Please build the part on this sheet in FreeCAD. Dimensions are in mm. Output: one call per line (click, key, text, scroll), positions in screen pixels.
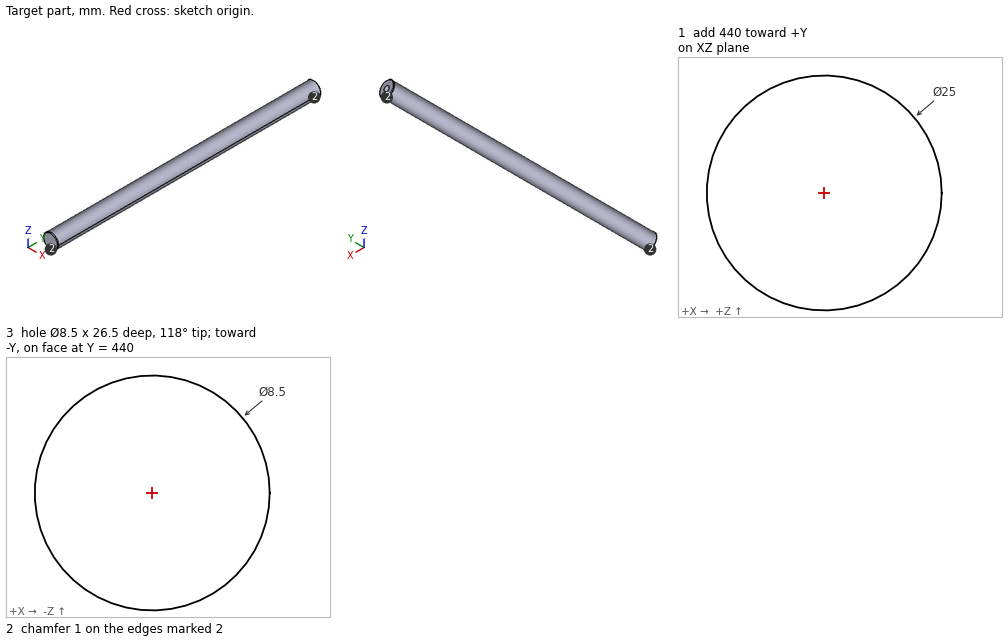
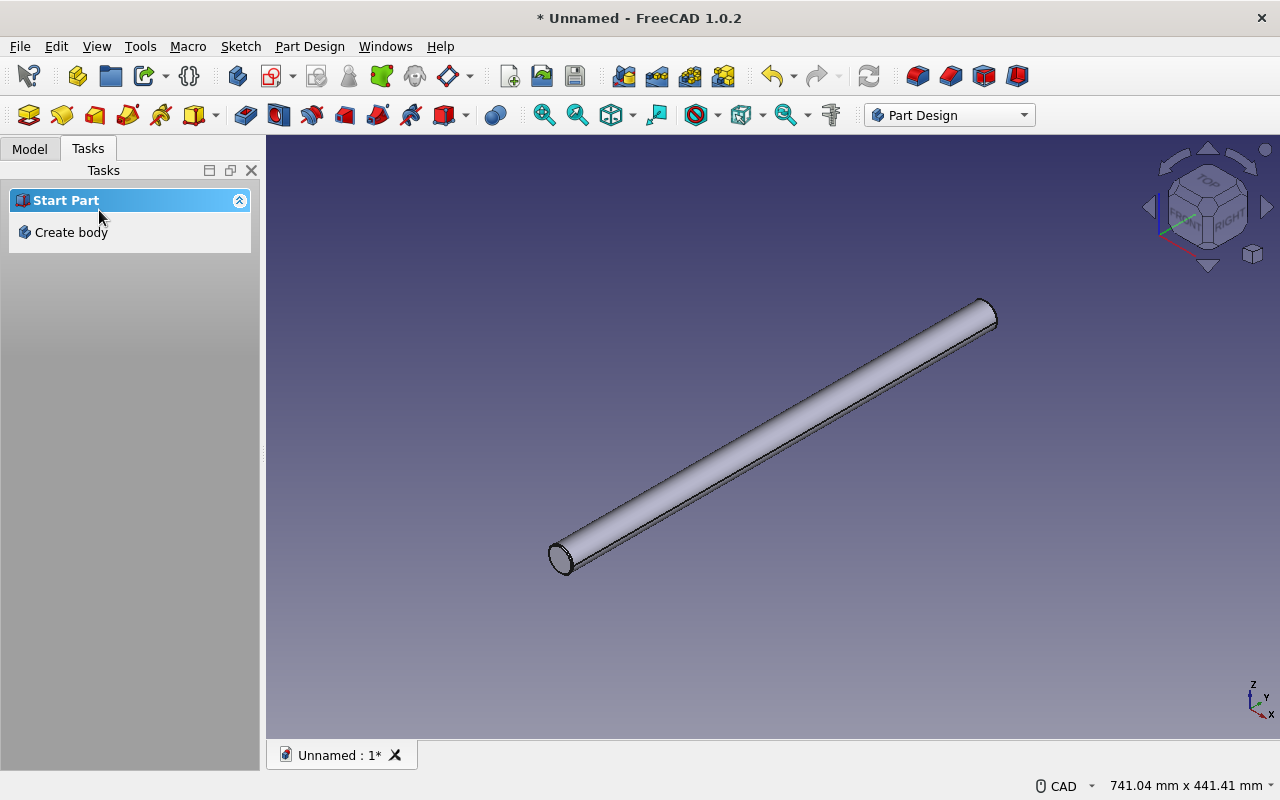
key(4)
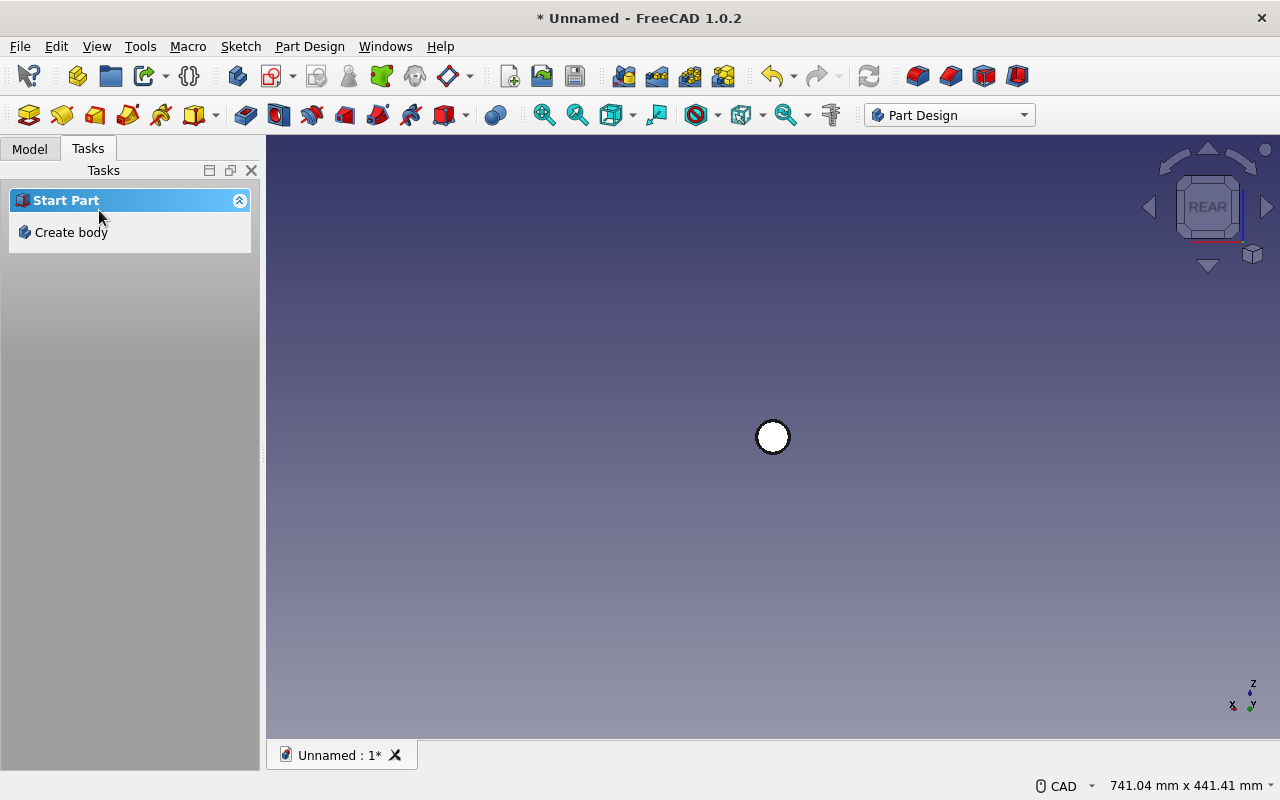
click(545, 116)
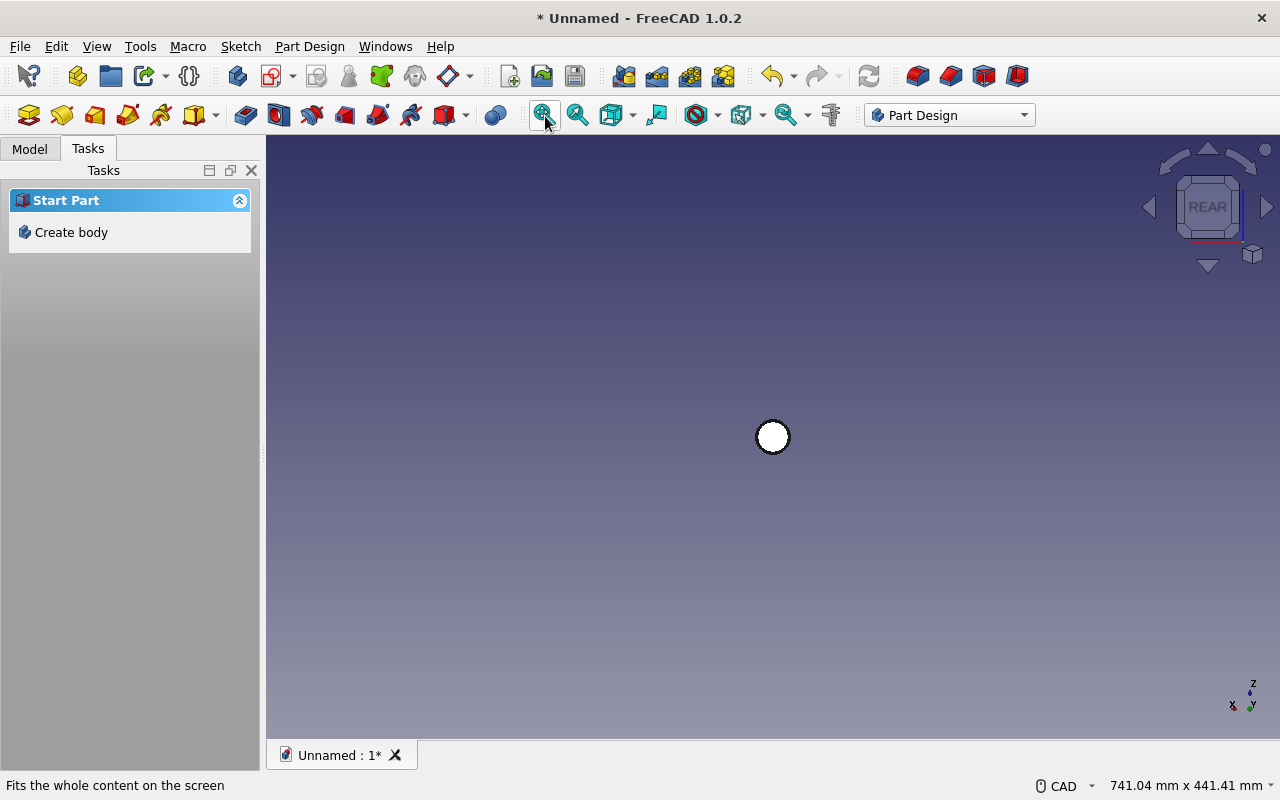
click(773, 436)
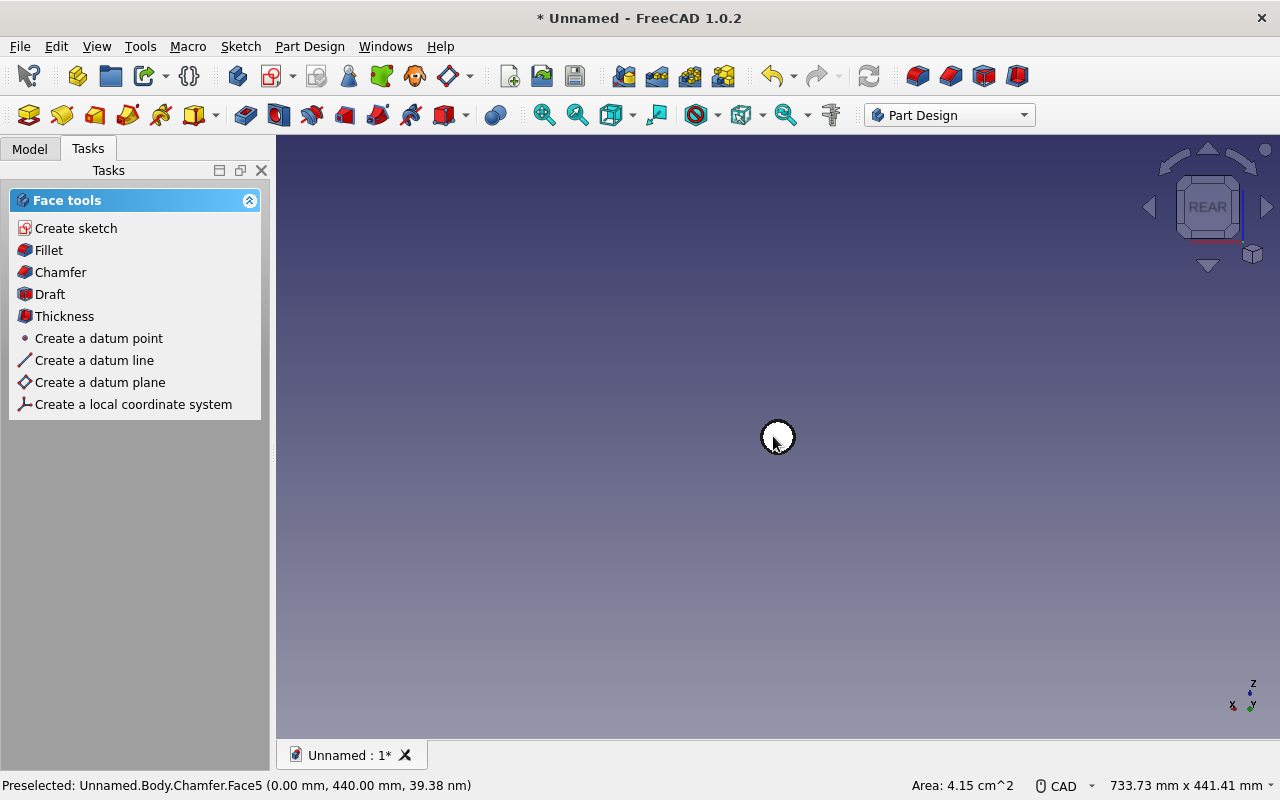
click(270, 76)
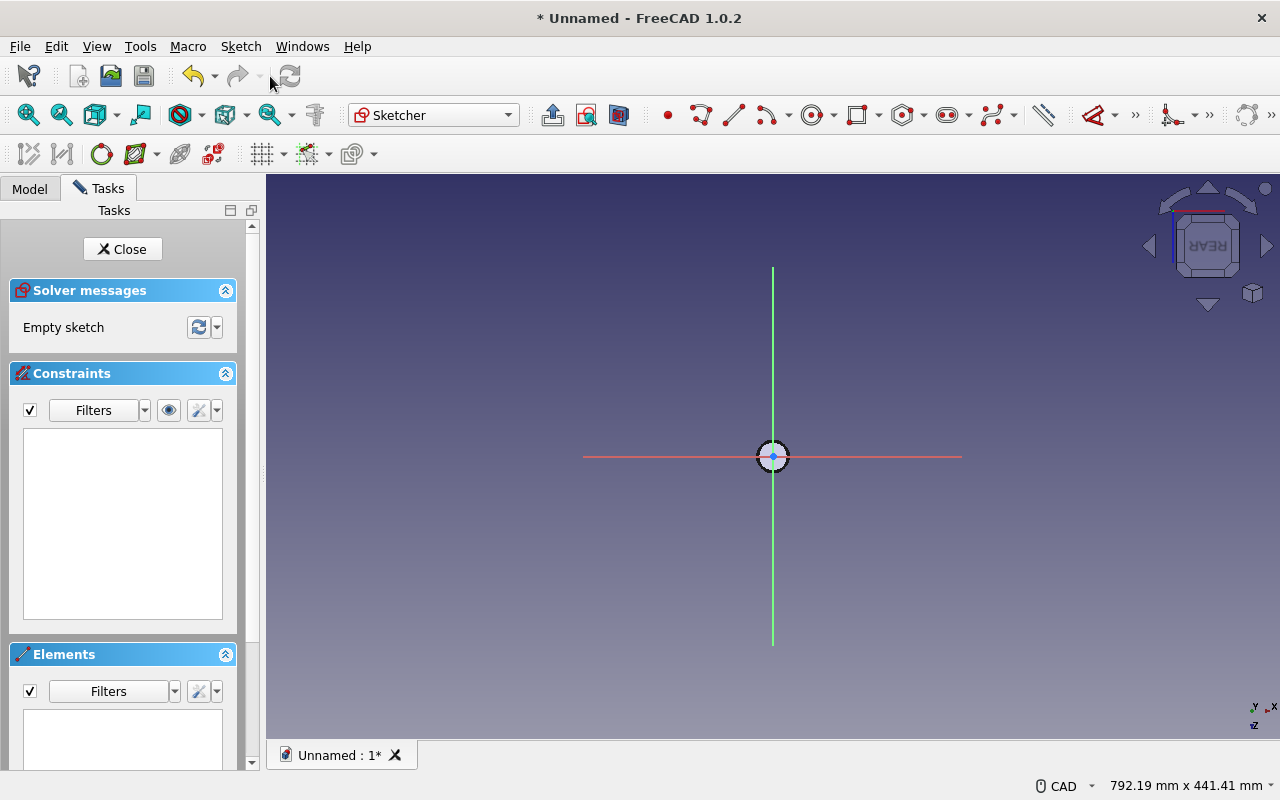
scroll(777, 456, up, 15)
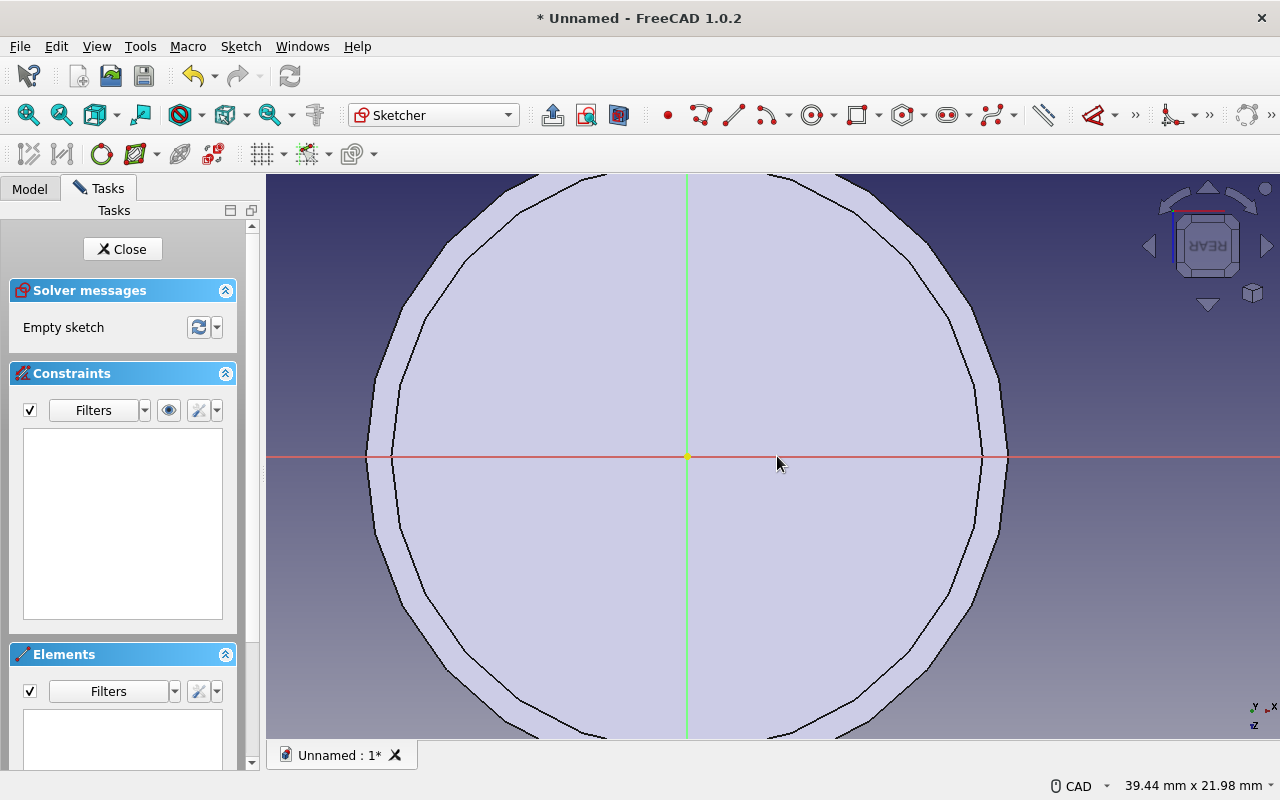
scroll(652, 456, up, 2)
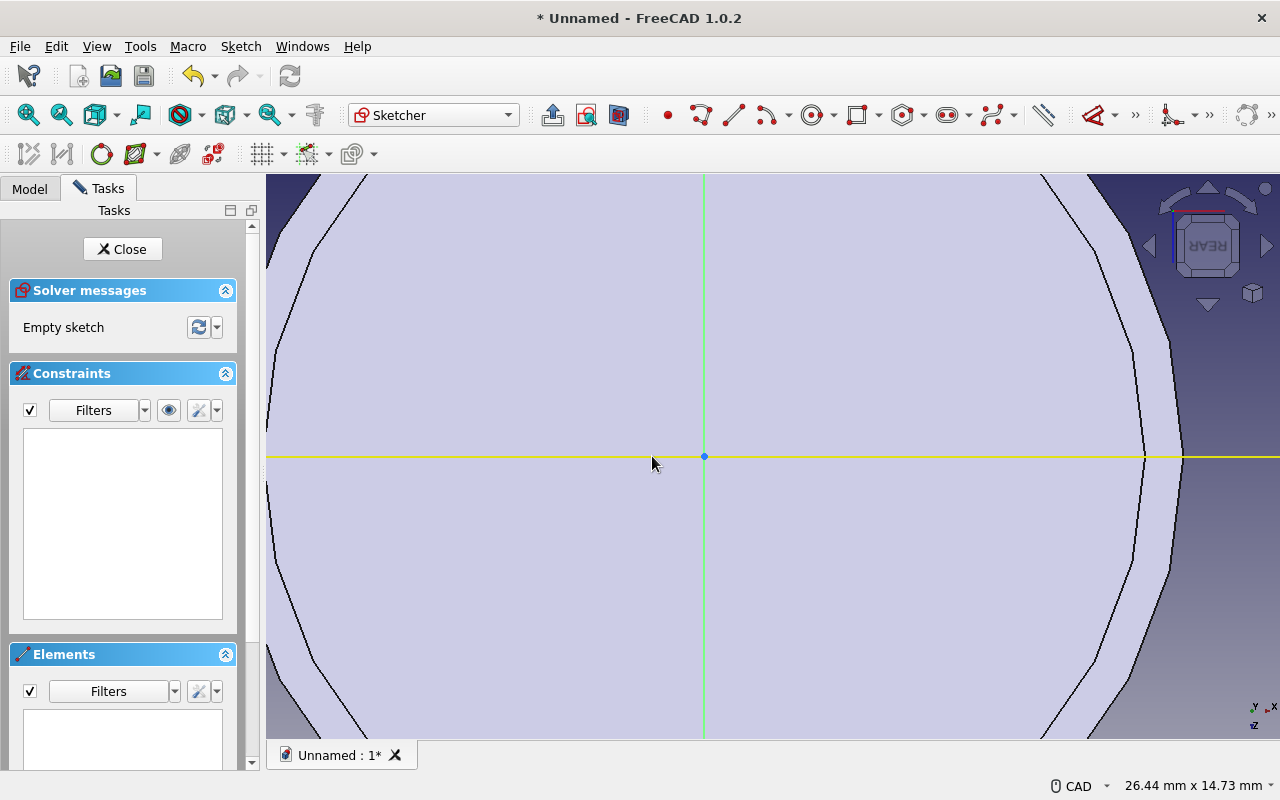
click(812, 116)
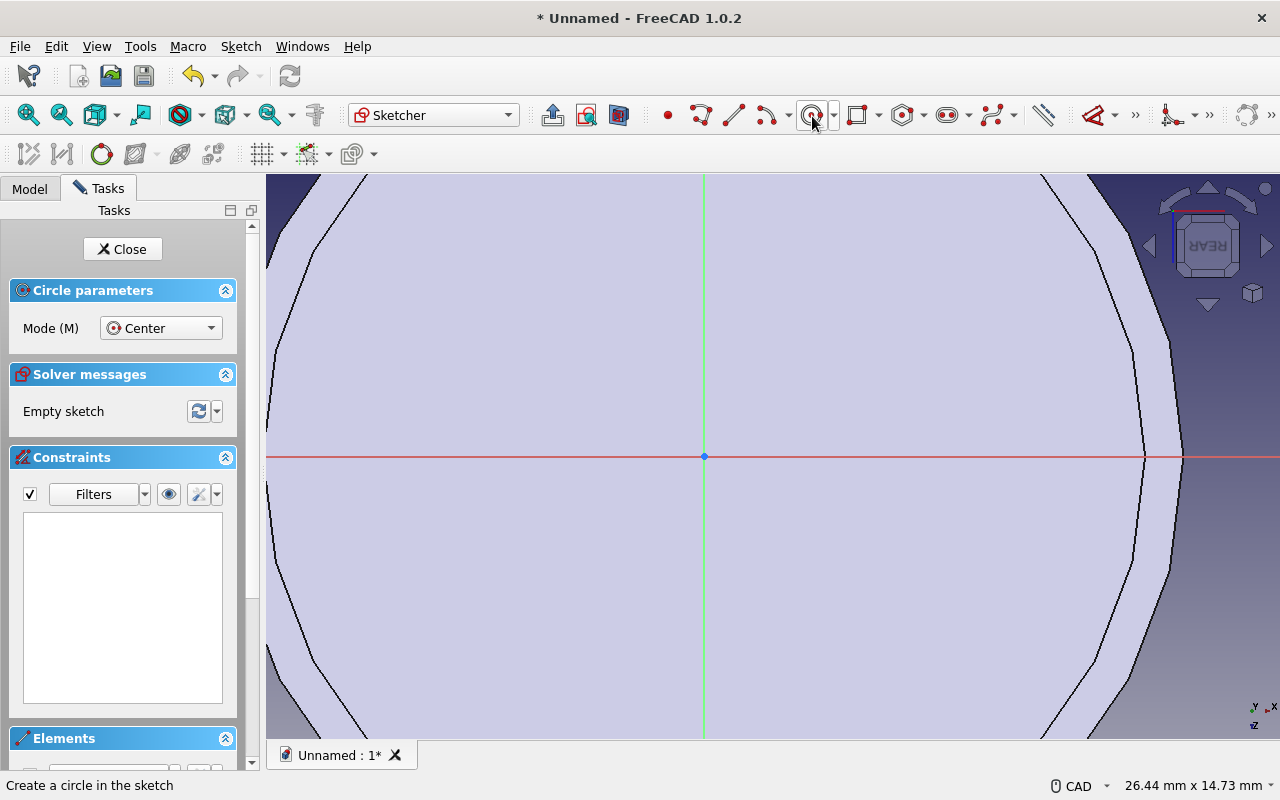
click(704, 456)
move(819, 341)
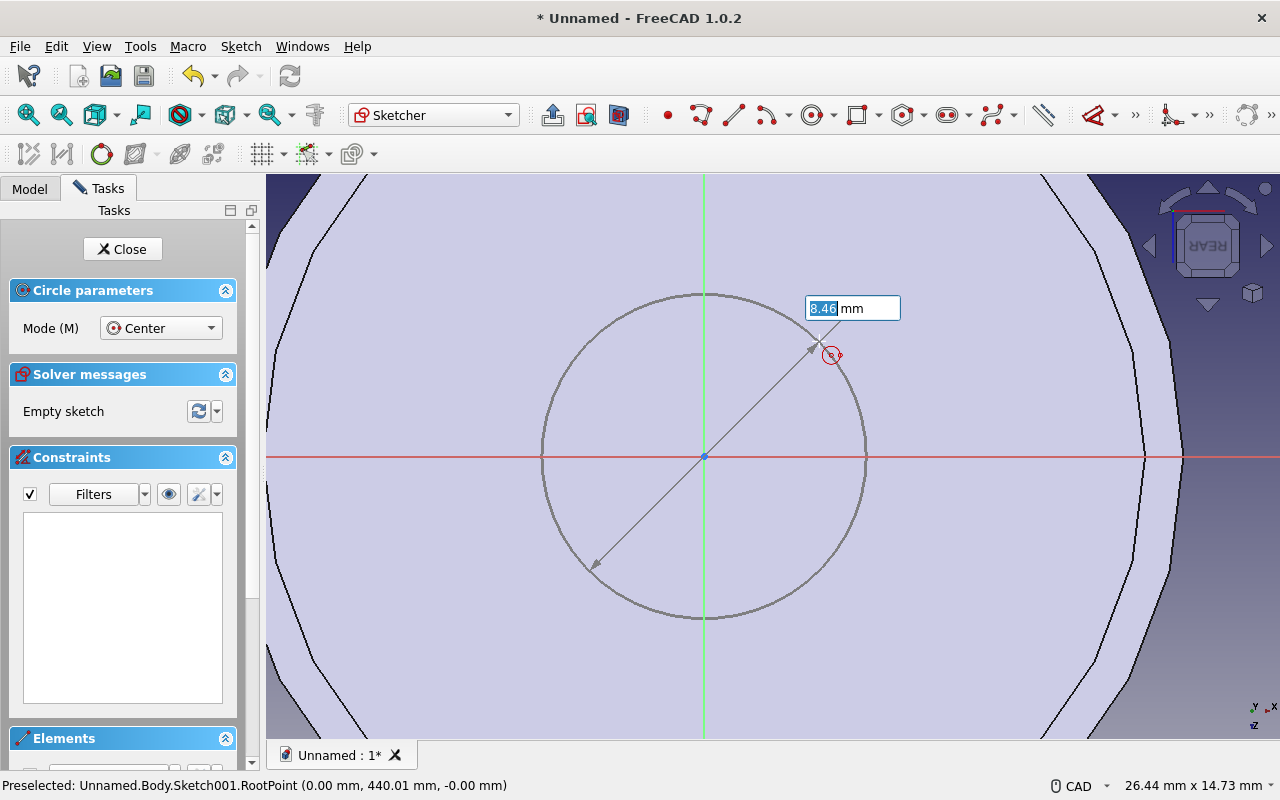
text(8.5)
key(Return)
key(Escape)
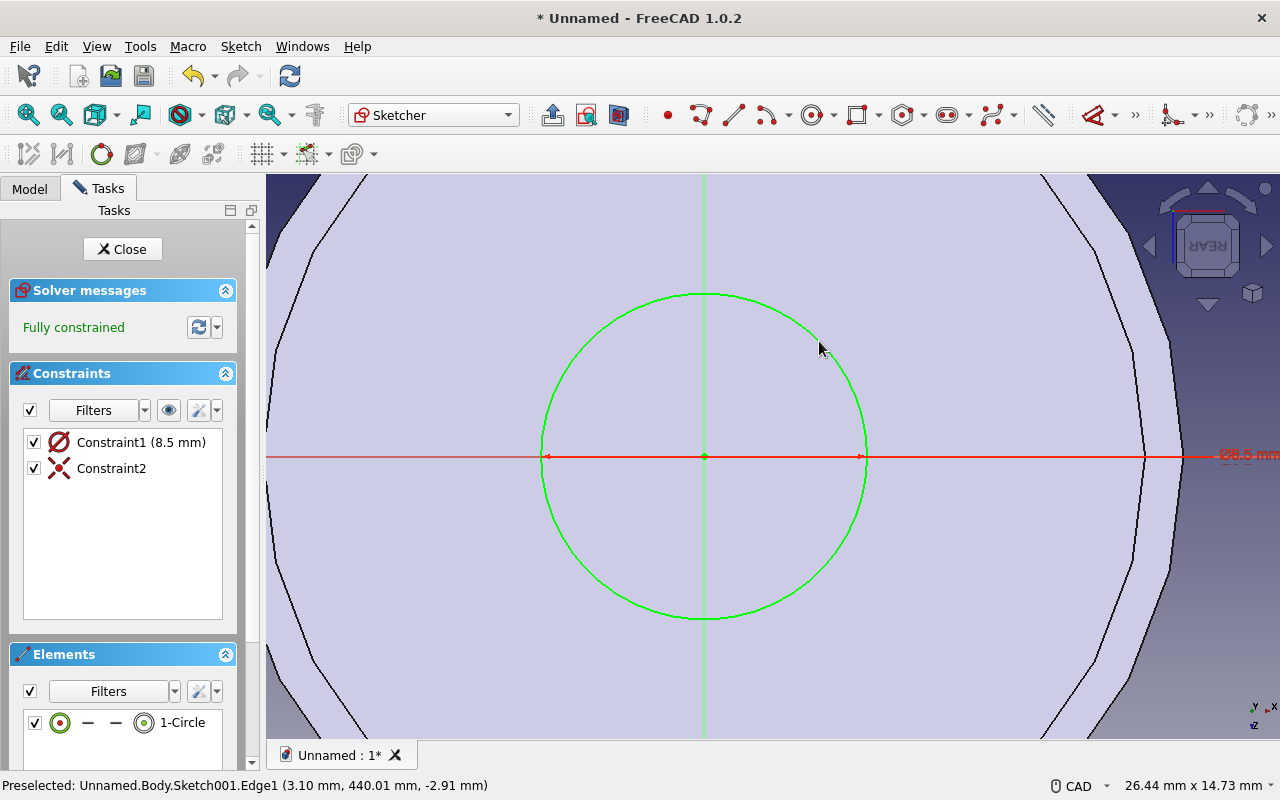
click(123, 249)